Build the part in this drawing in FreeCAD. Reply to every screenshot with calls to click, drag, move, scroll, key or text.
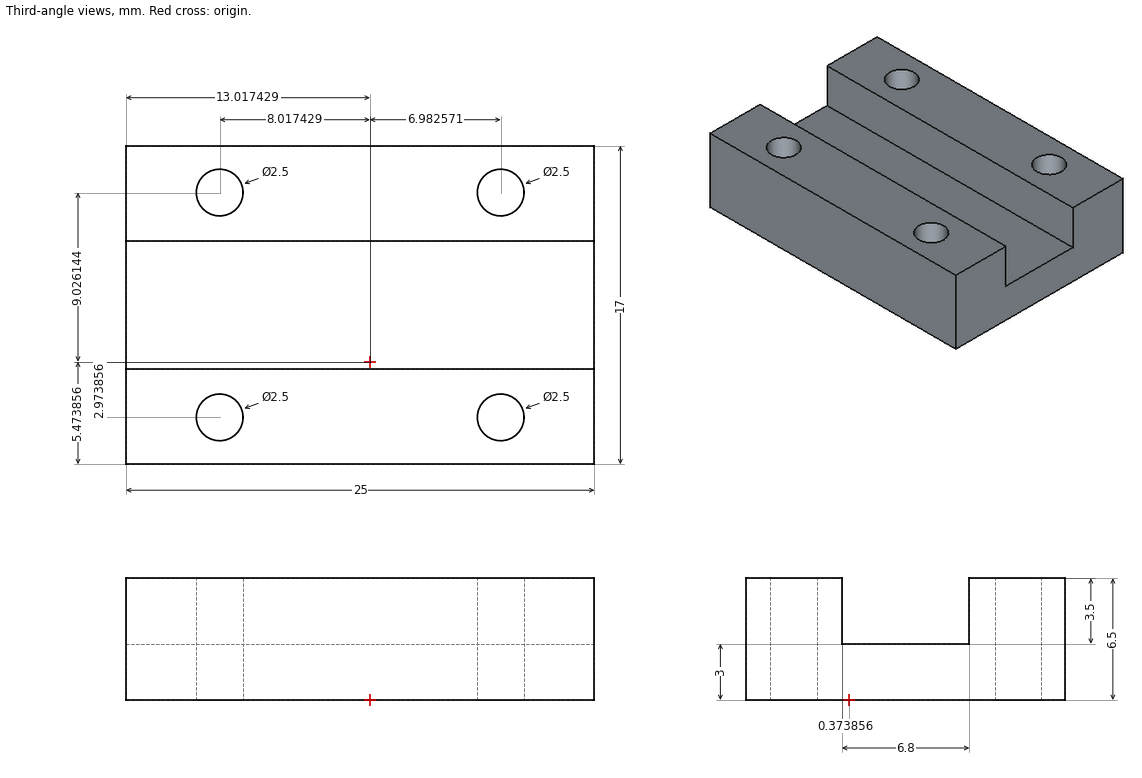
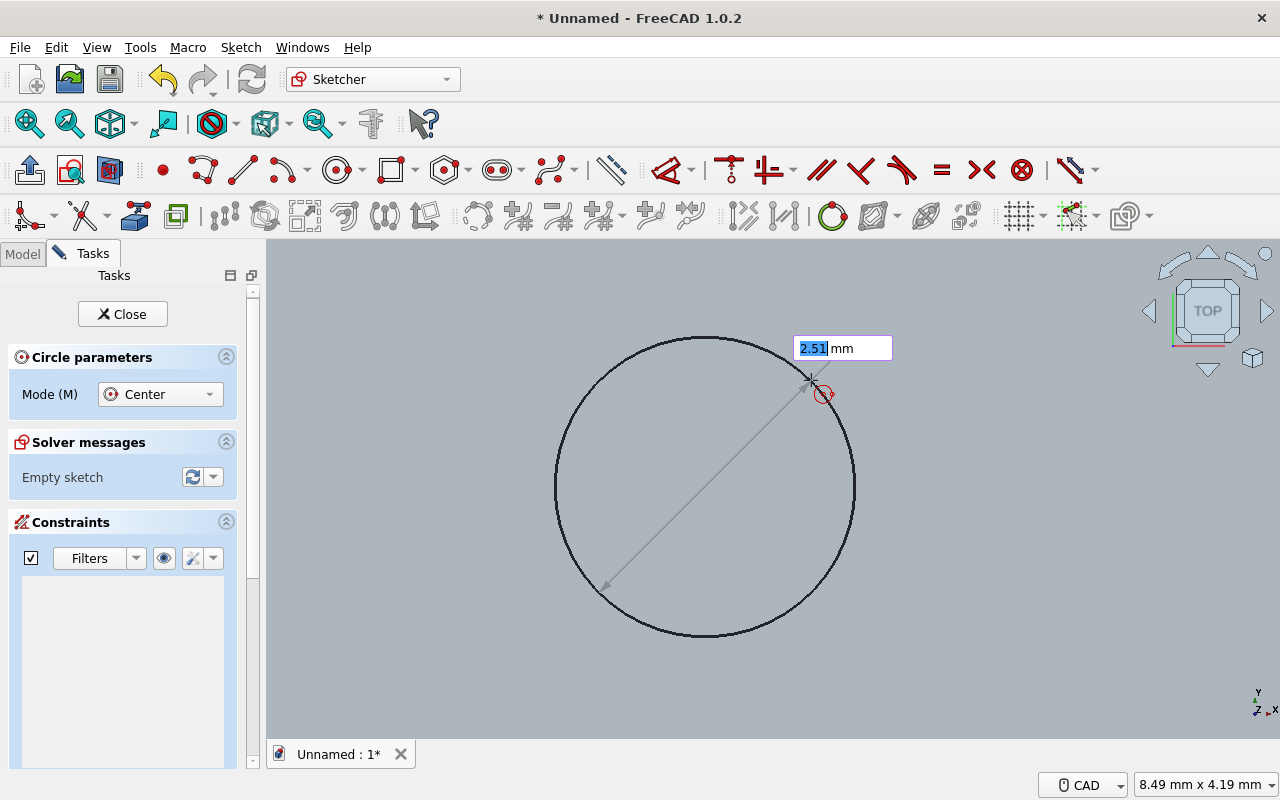
text(2.5)
key(Return)
key(Escape)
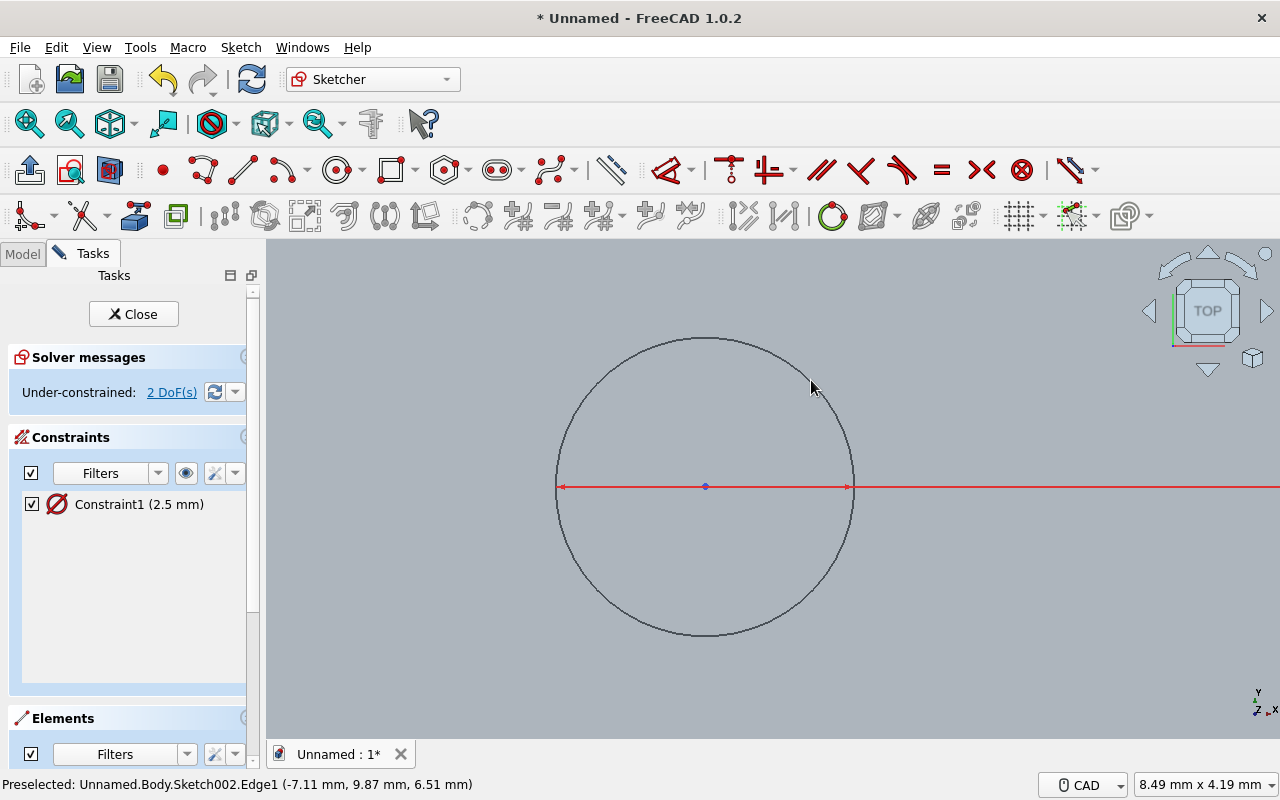
key(d)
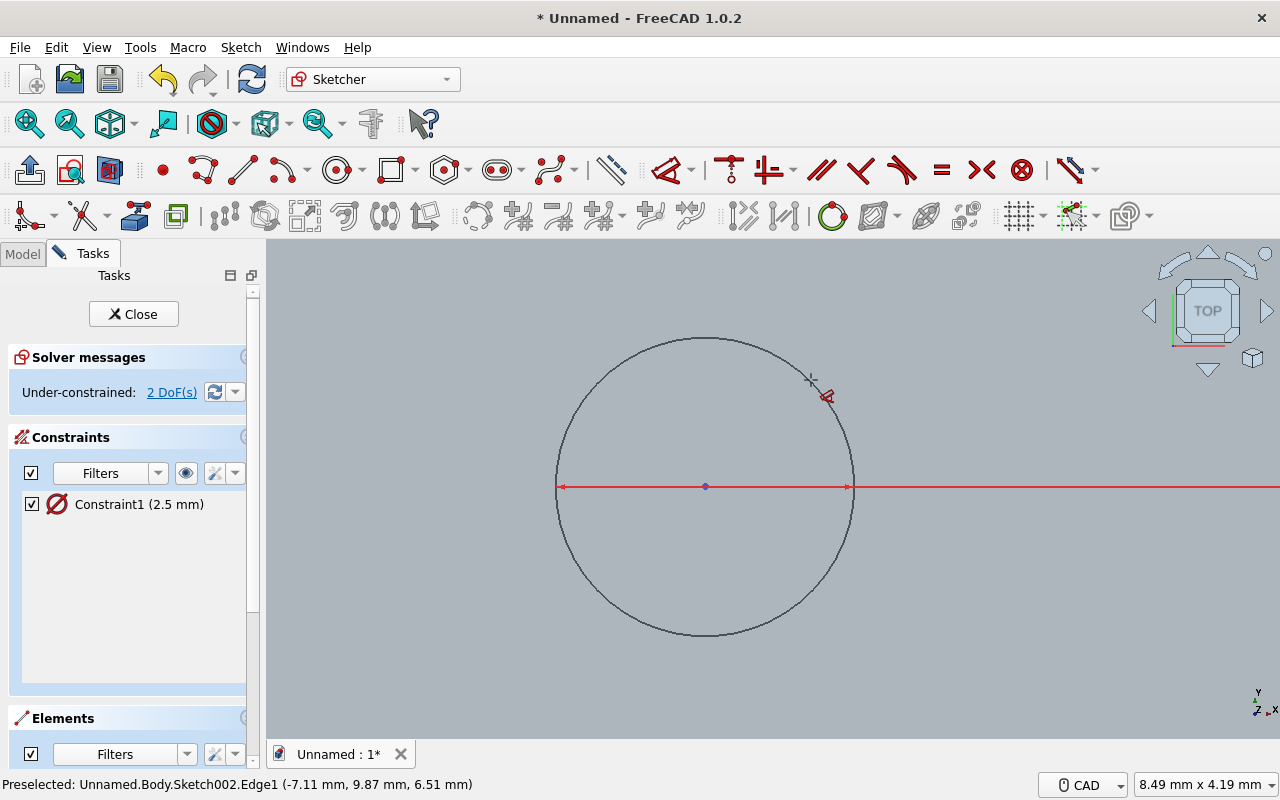
click(705, 487)
click(910, 453)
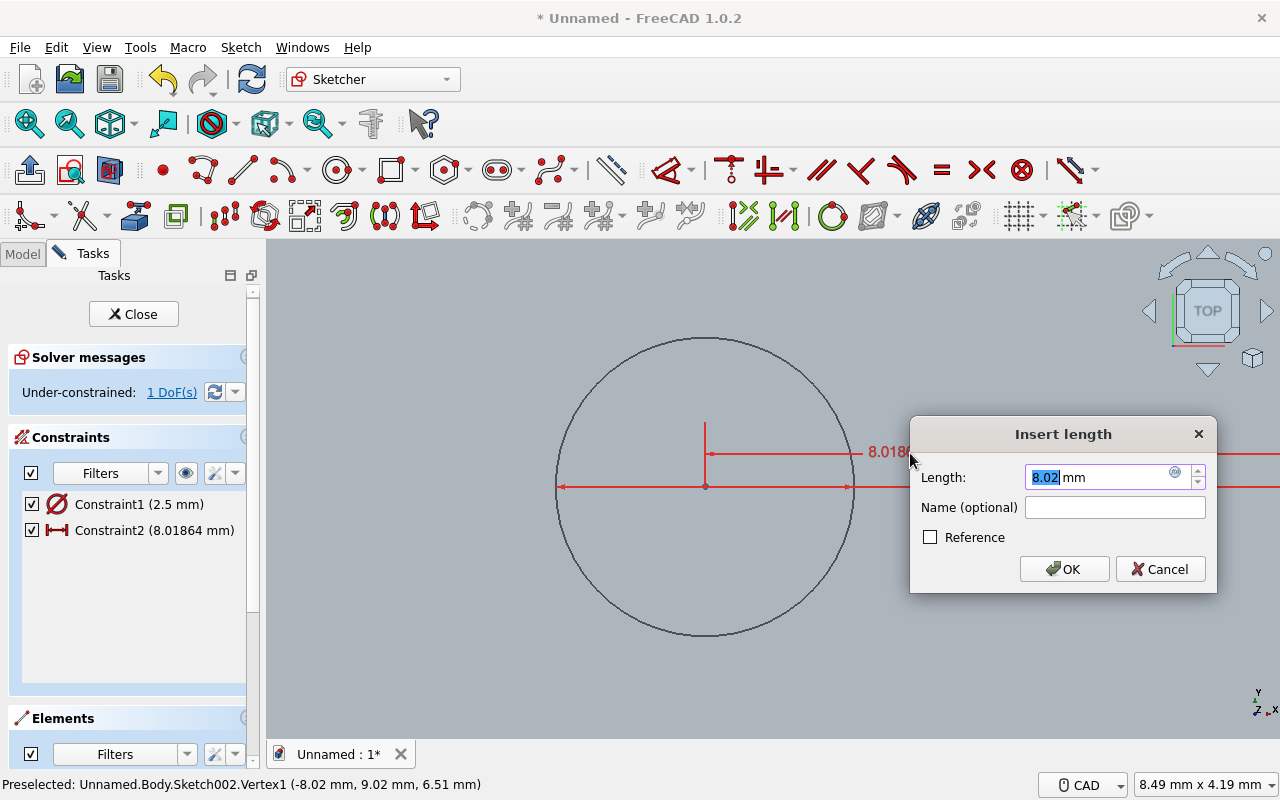
text(8.017429)
key(Return)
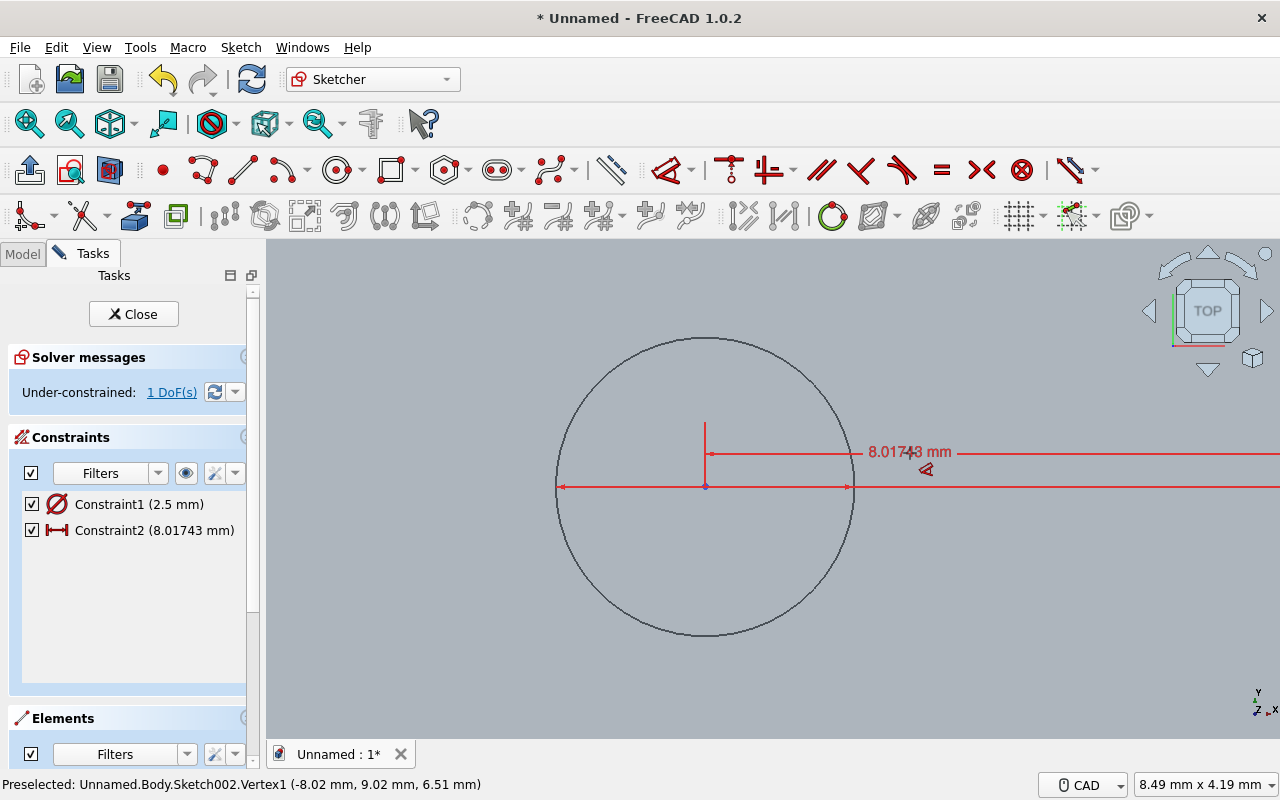
click(705, 487)
click(671, 599)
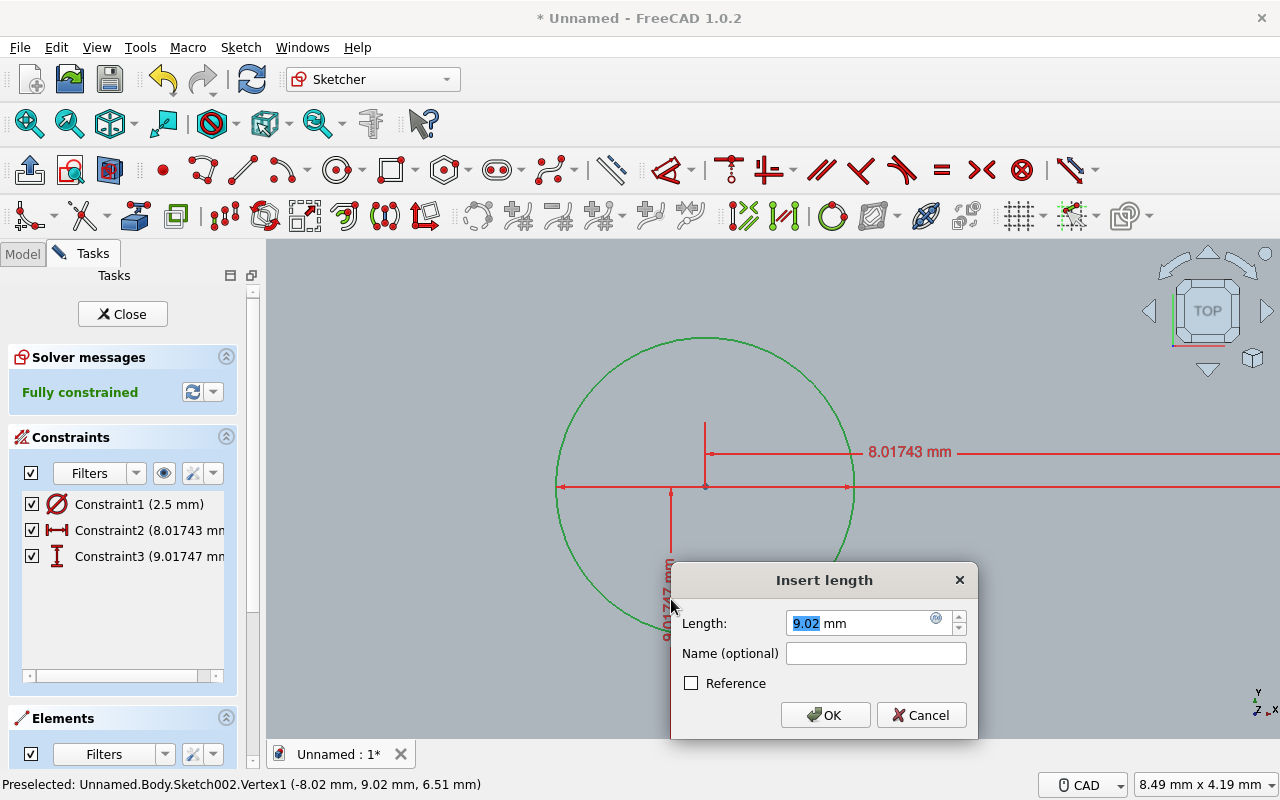
text(9.026144)
key(Return)
key(Escape)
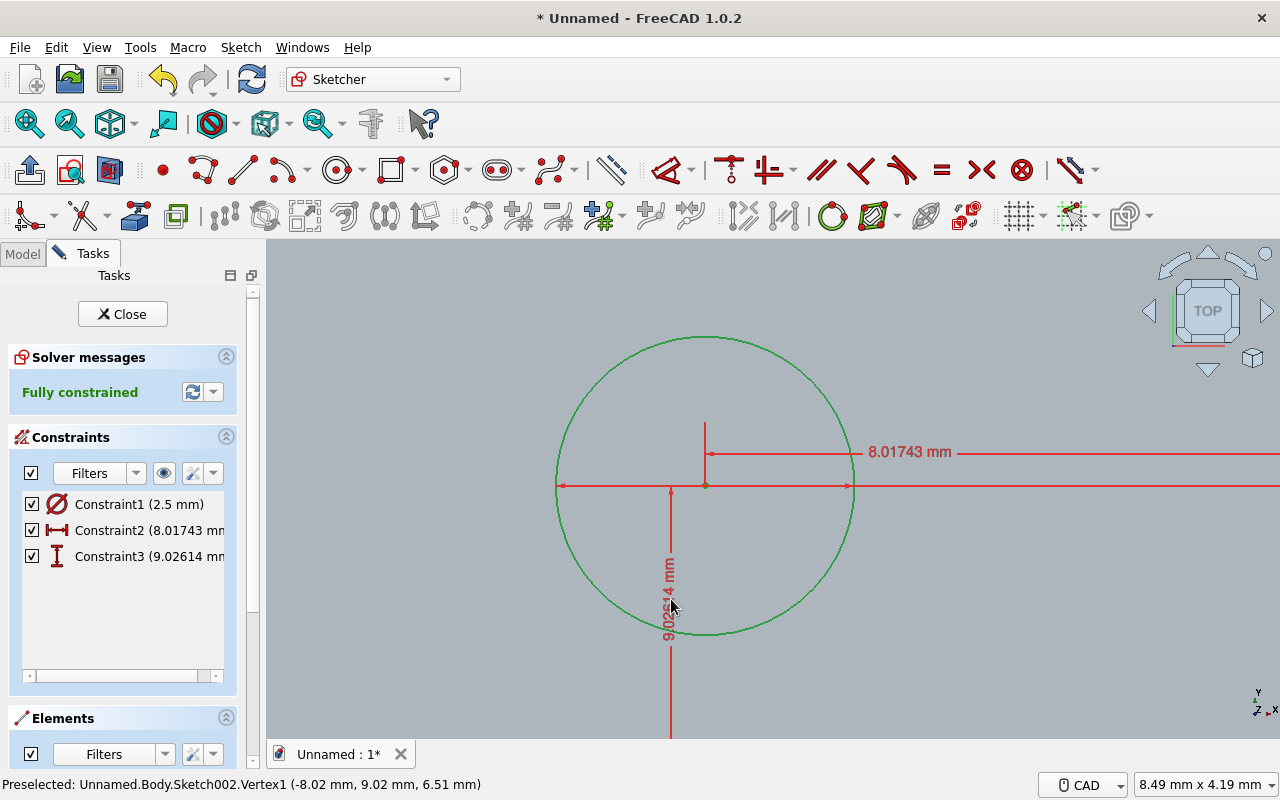
click(123, 314)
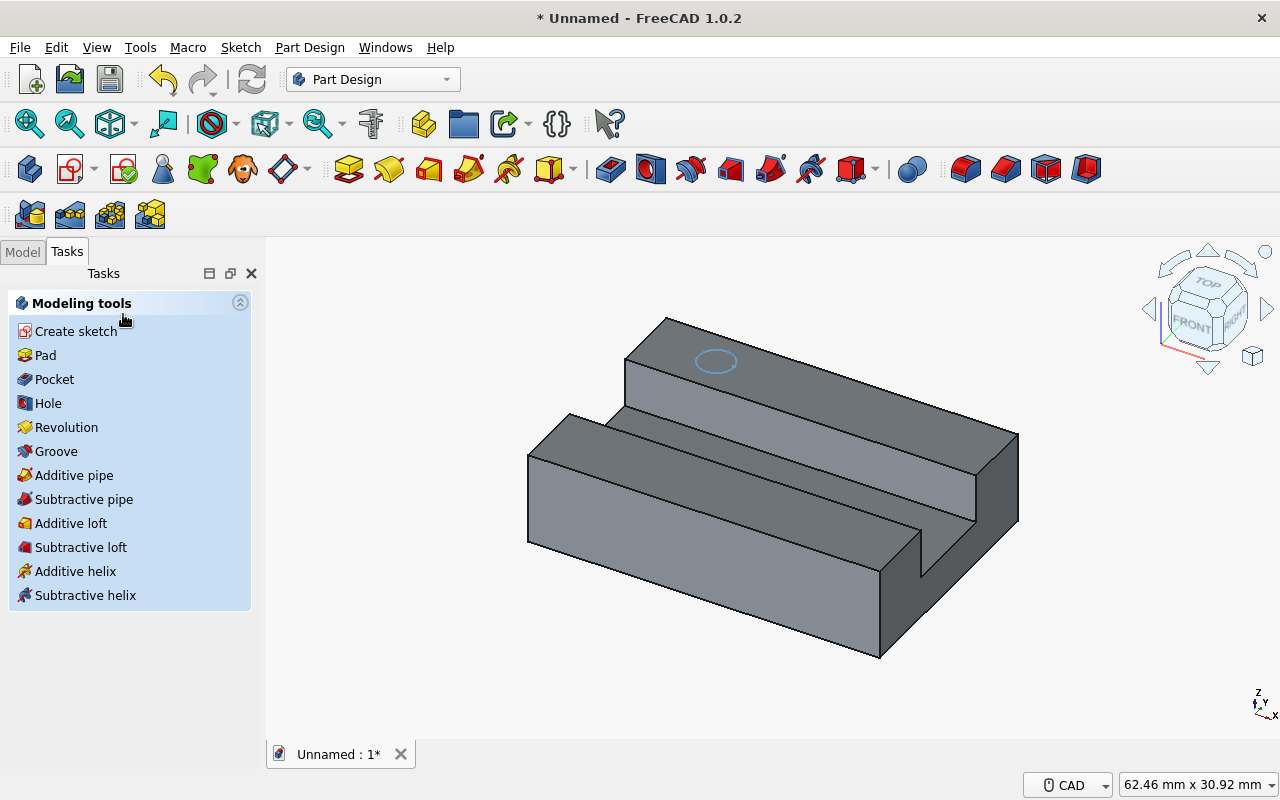
click(612, 170)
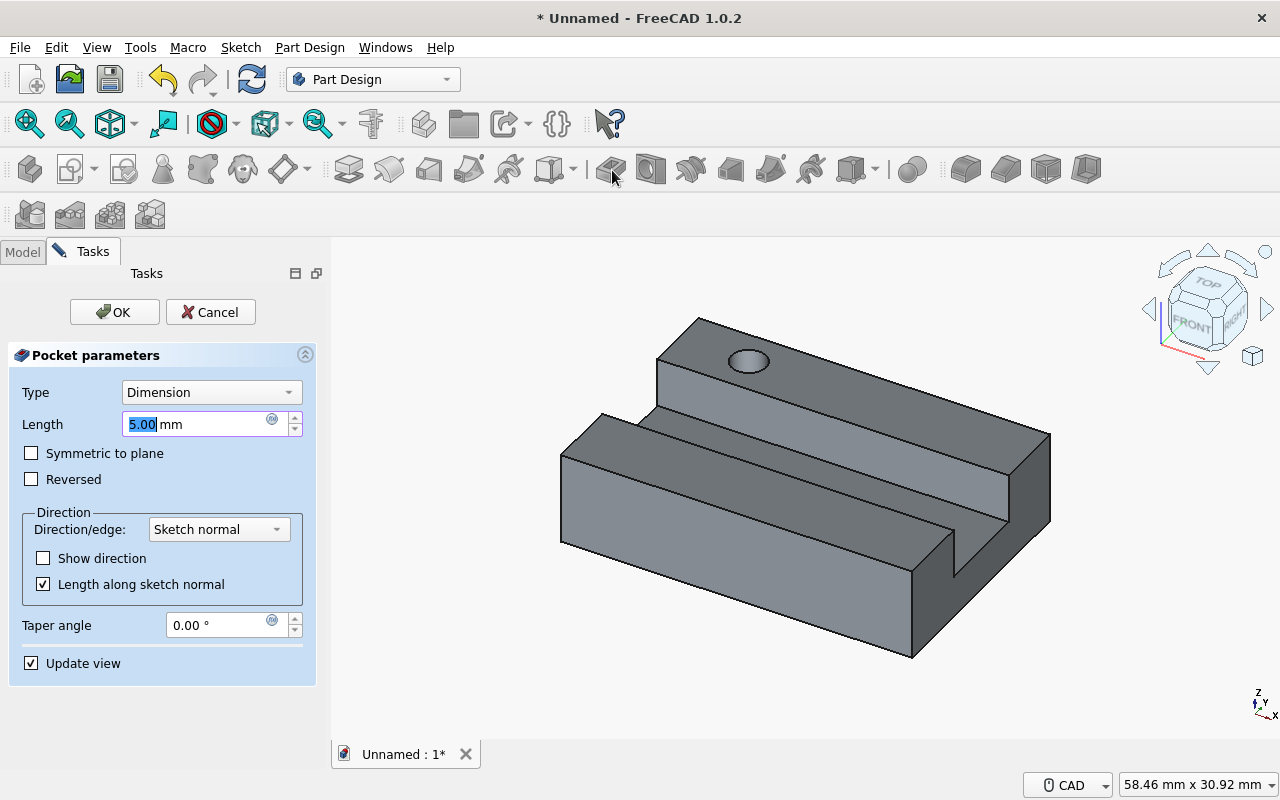
click(212, 392)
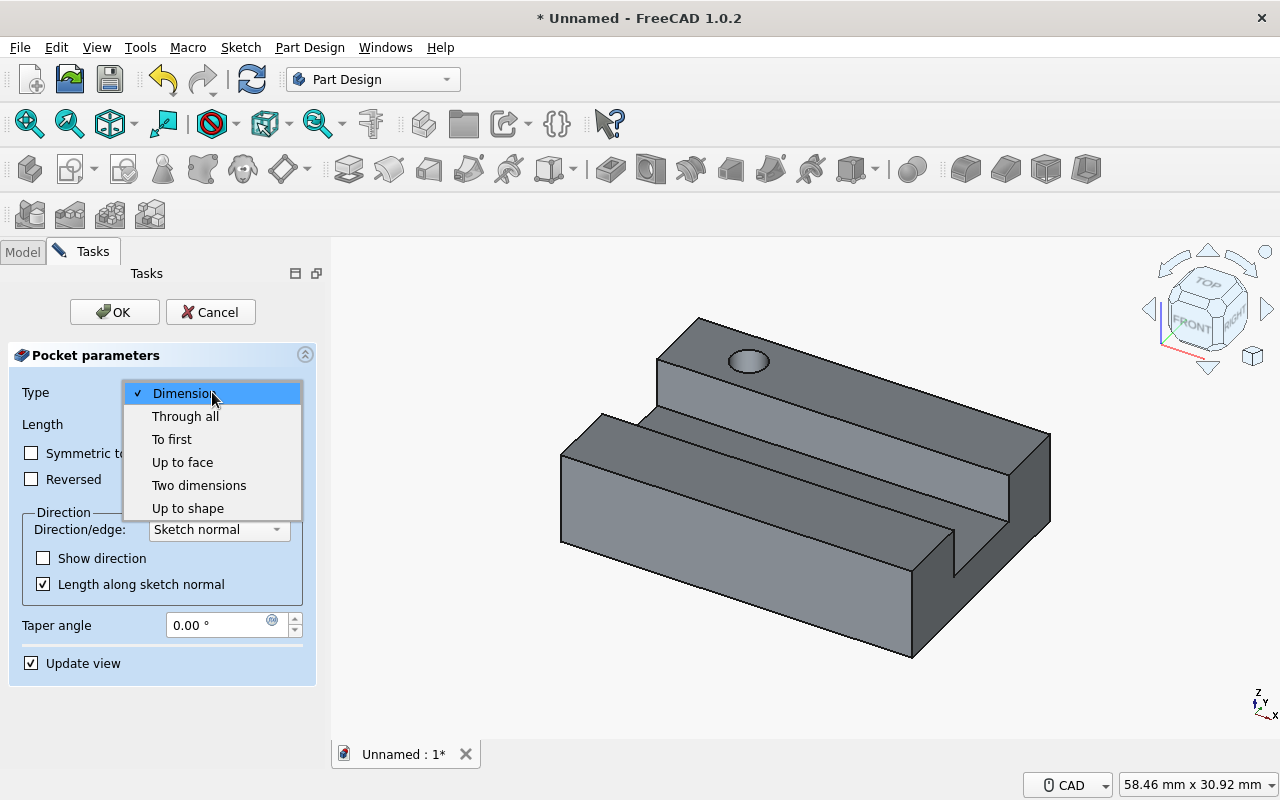
click(212, 440)